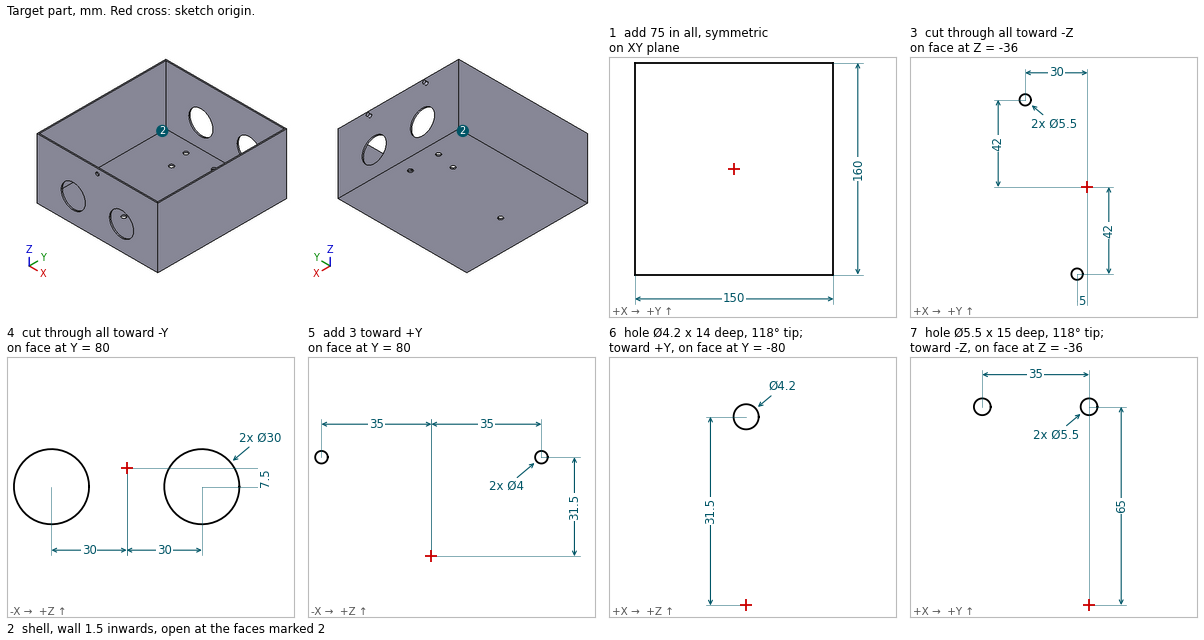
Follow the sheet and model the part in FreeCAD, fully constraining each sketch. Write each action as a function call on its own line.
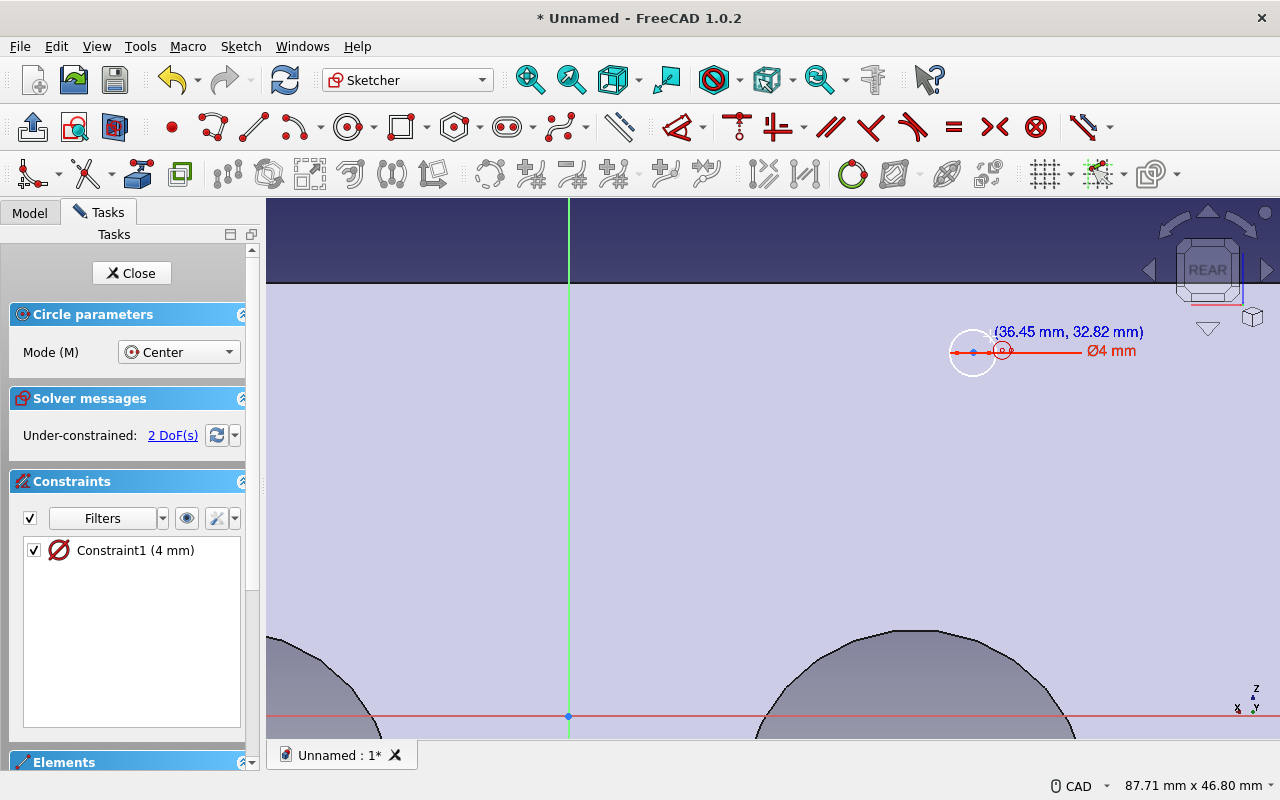
scroll(981, 358, down, 2)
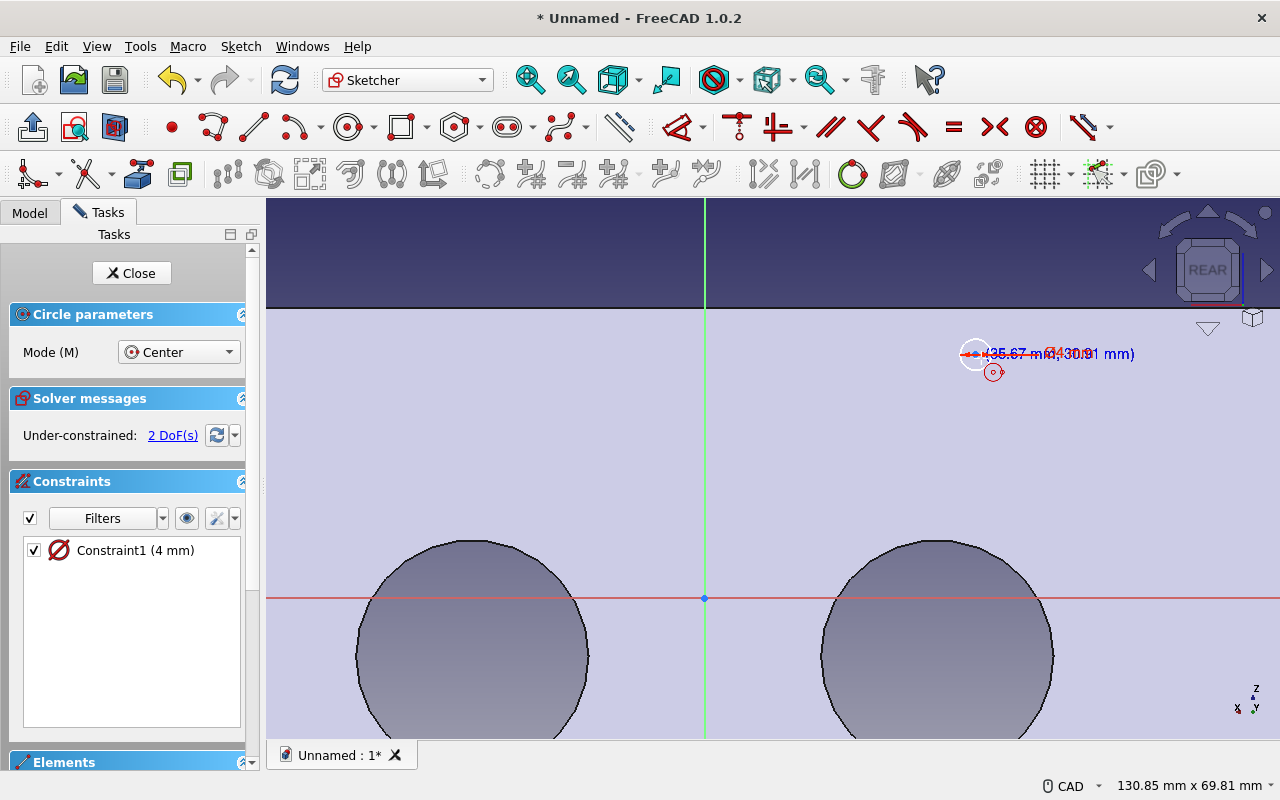
scroll(434, 354, up, 2)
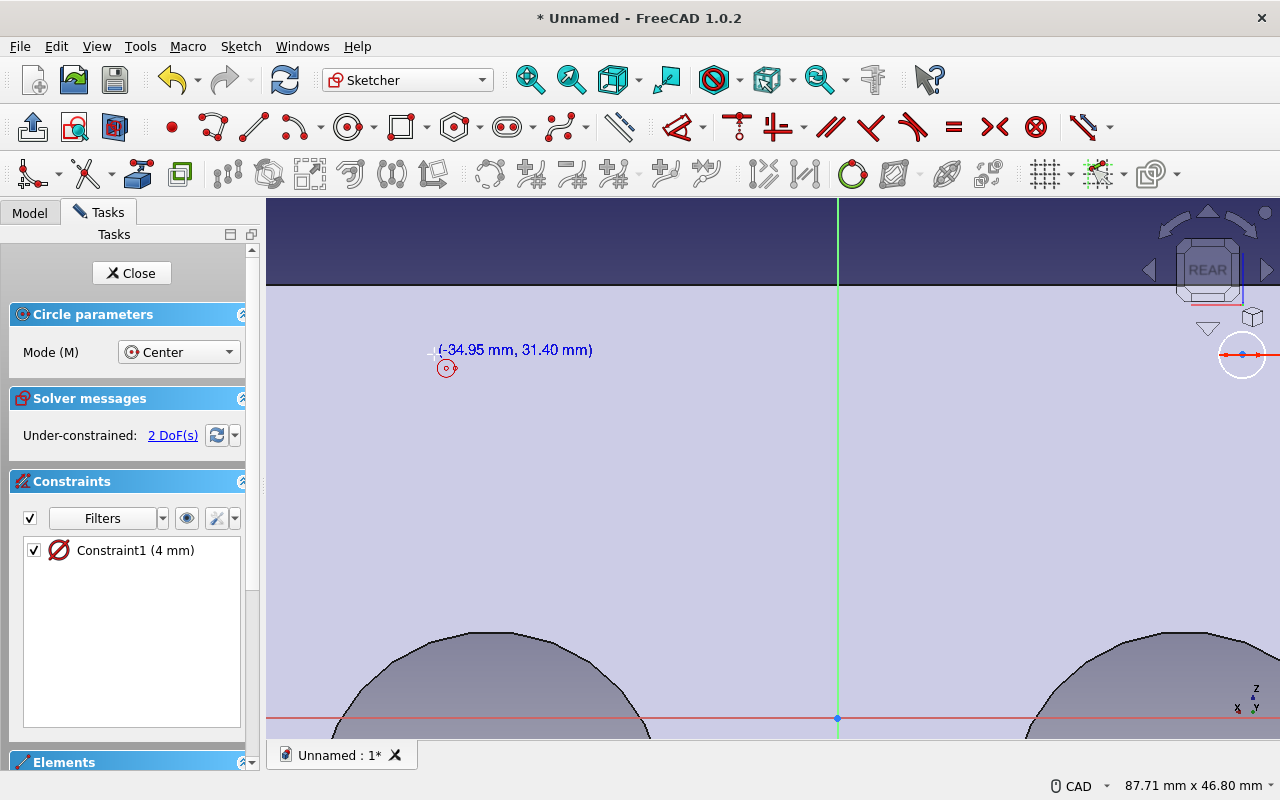
click(433, 354)
move(450, 338)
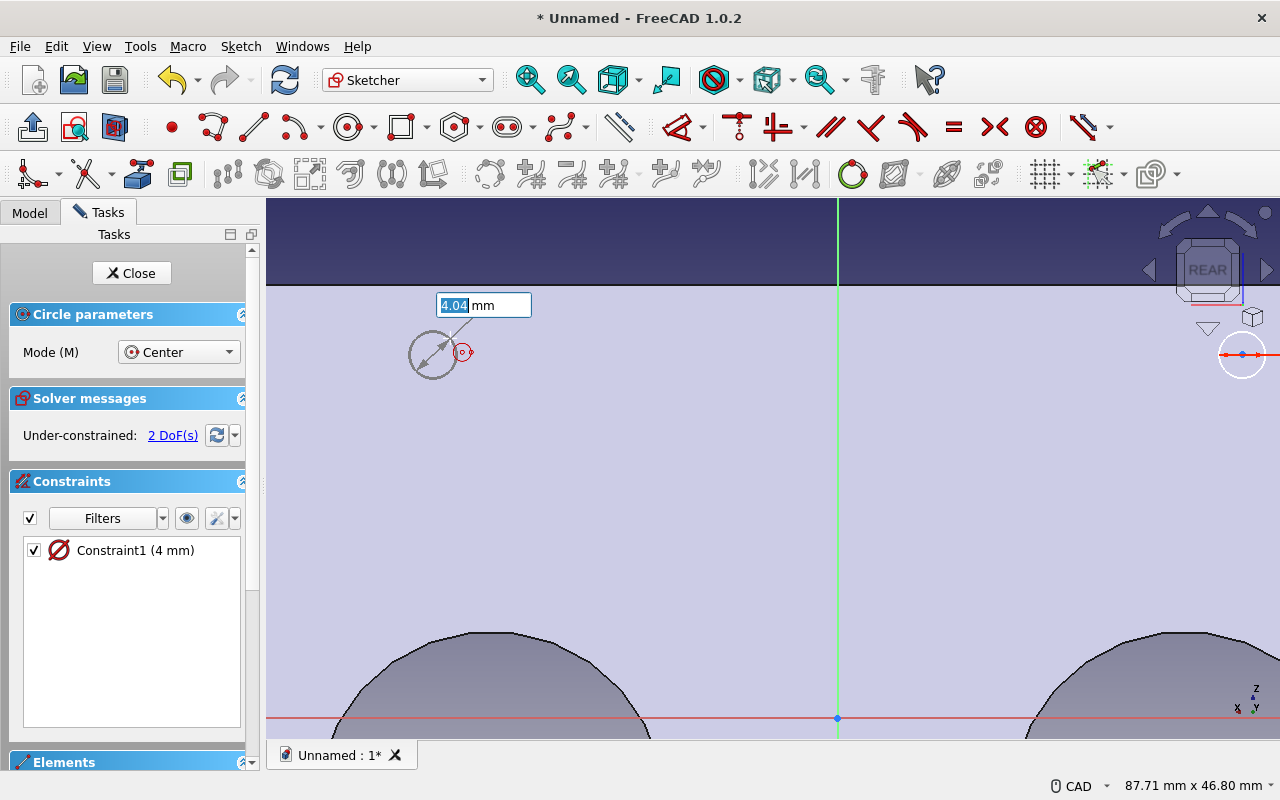
text(4)
key(Return)
key(Escape)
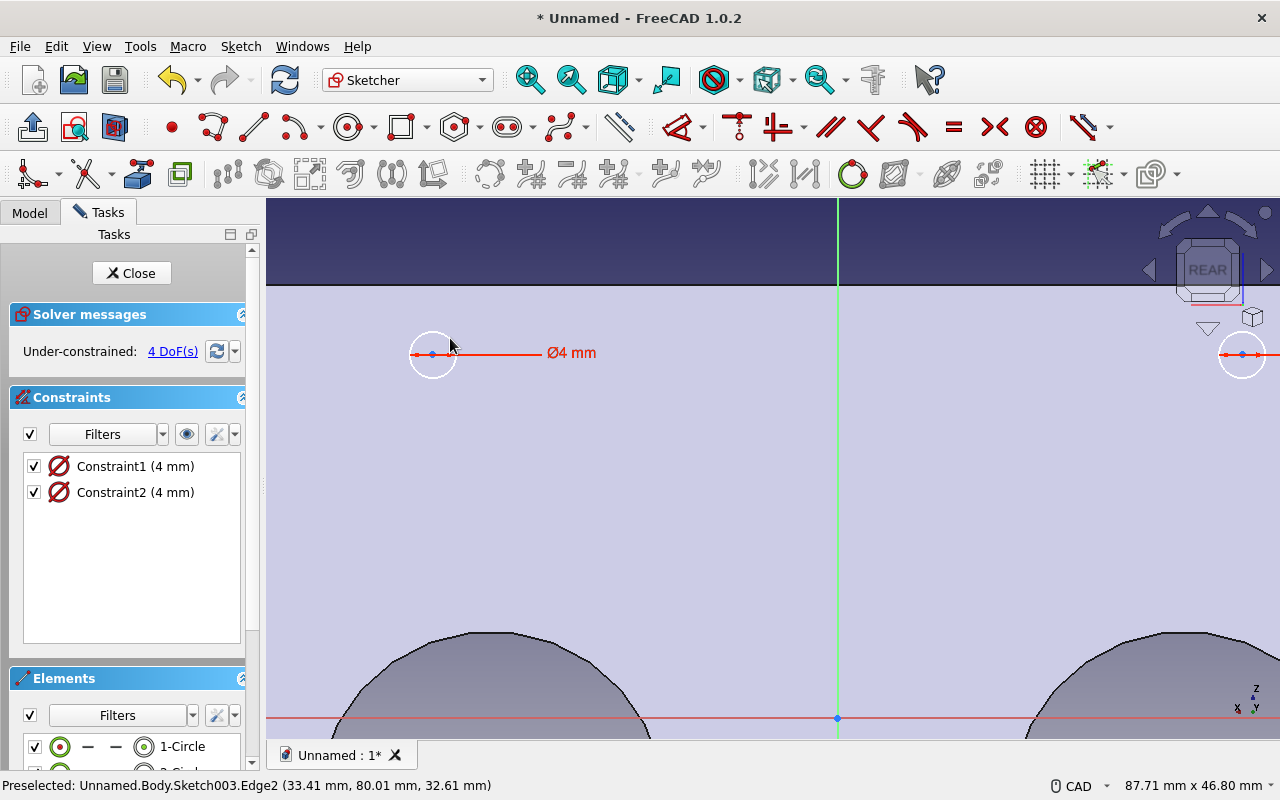
scroll(433, 354, down, 2)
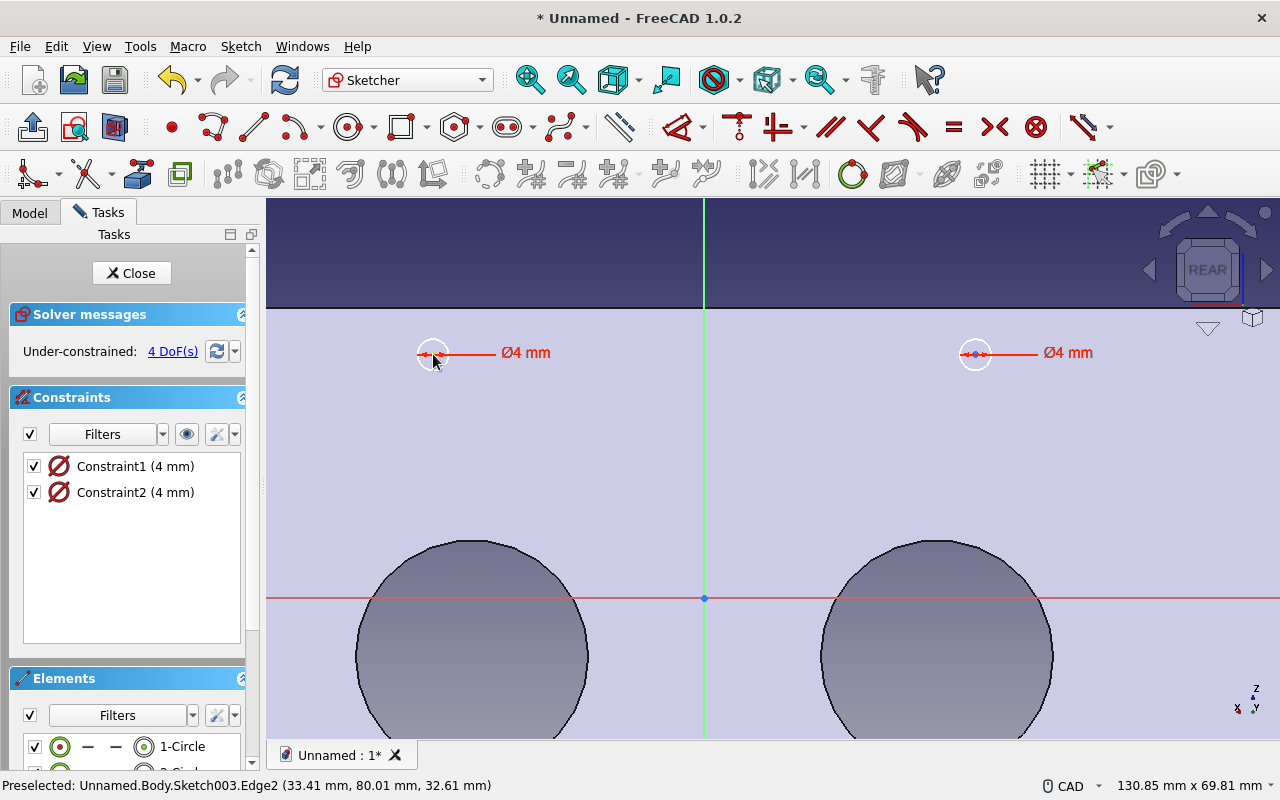
click(976, 355)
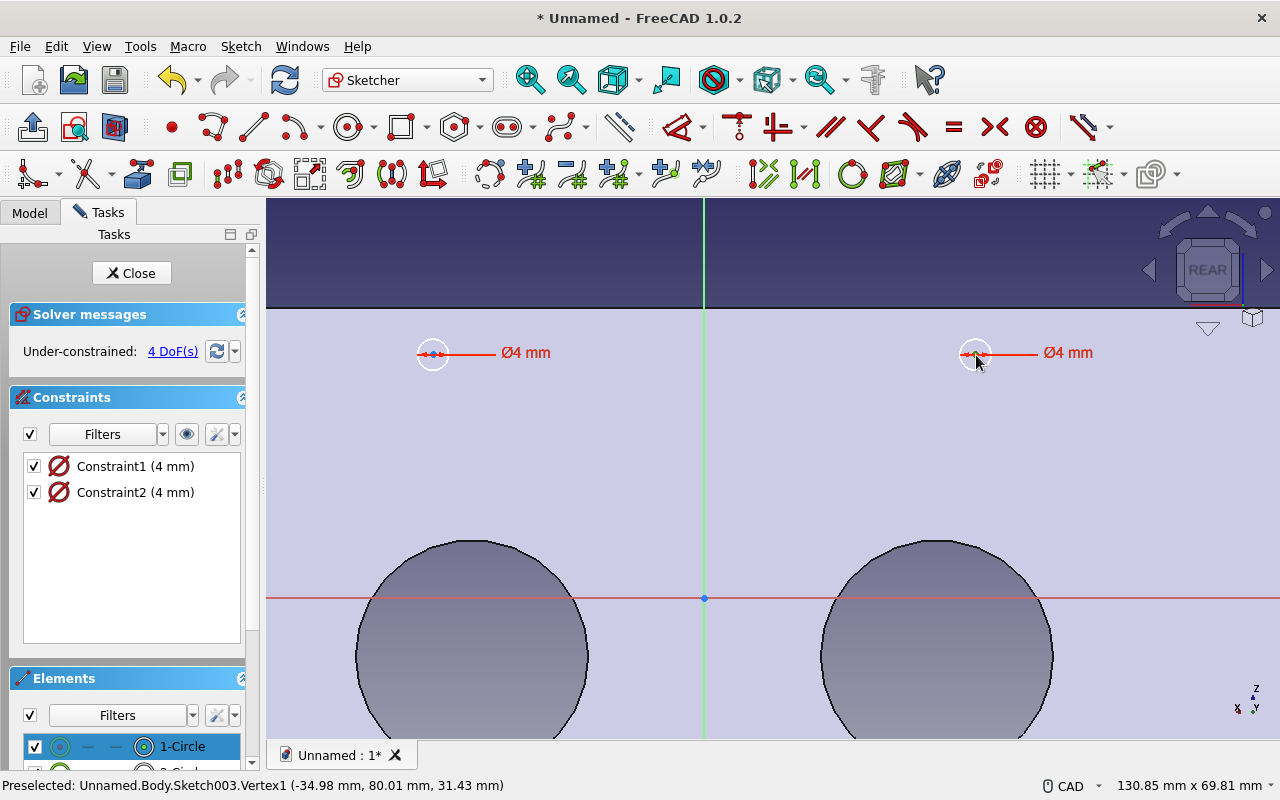
click(433, 355)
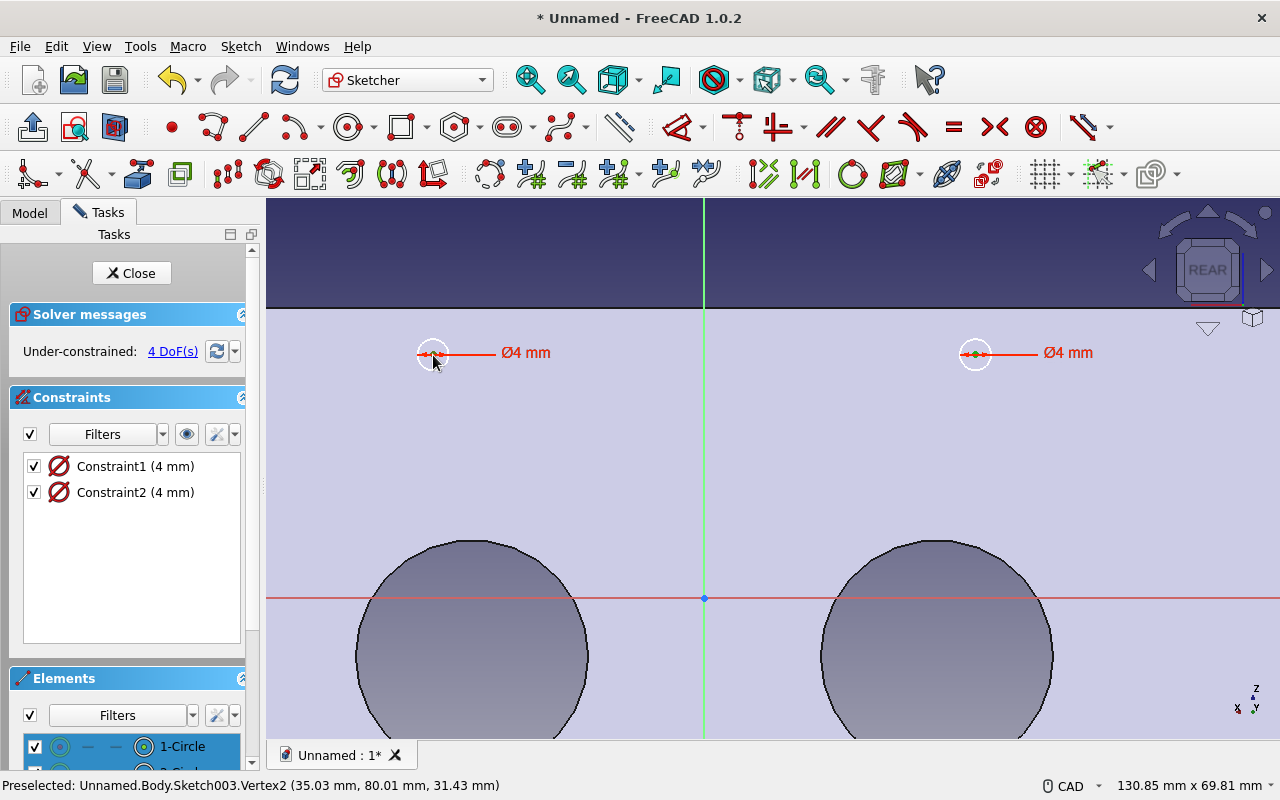
key(h)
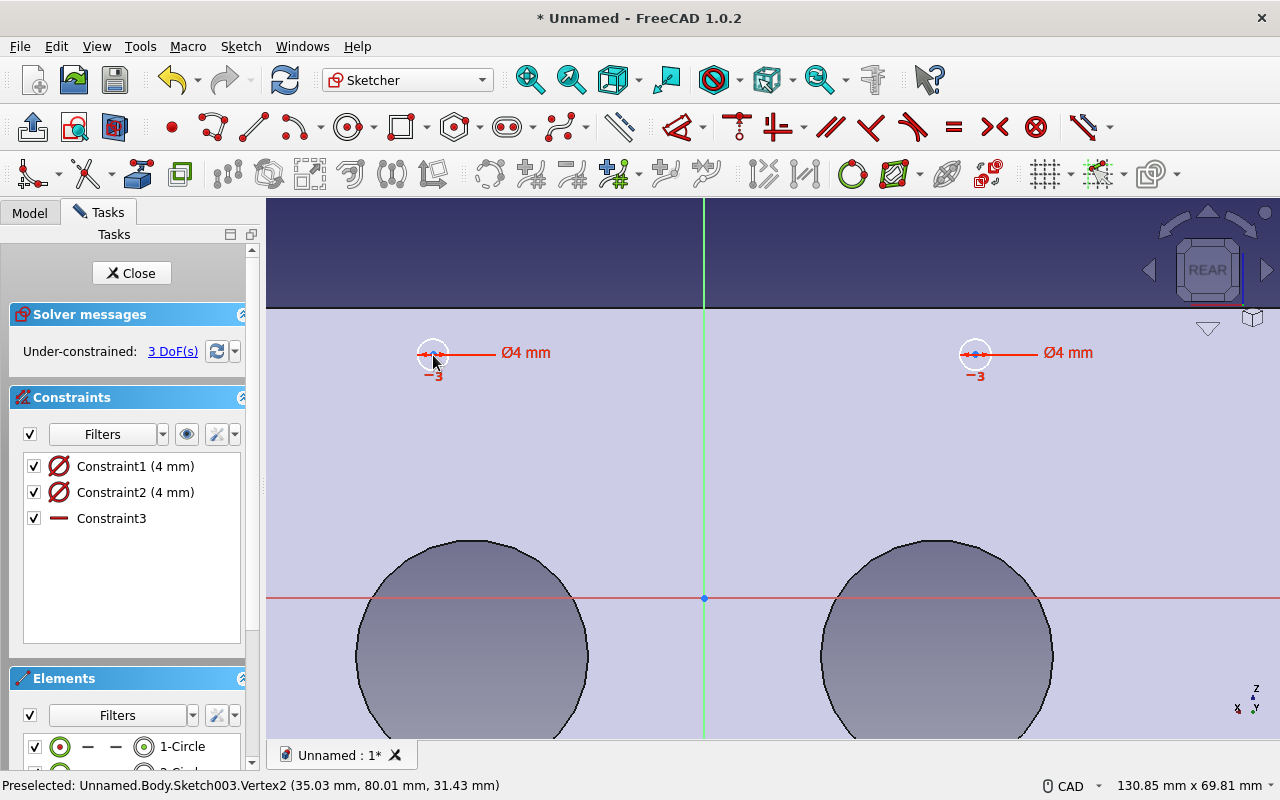
click(676, 128)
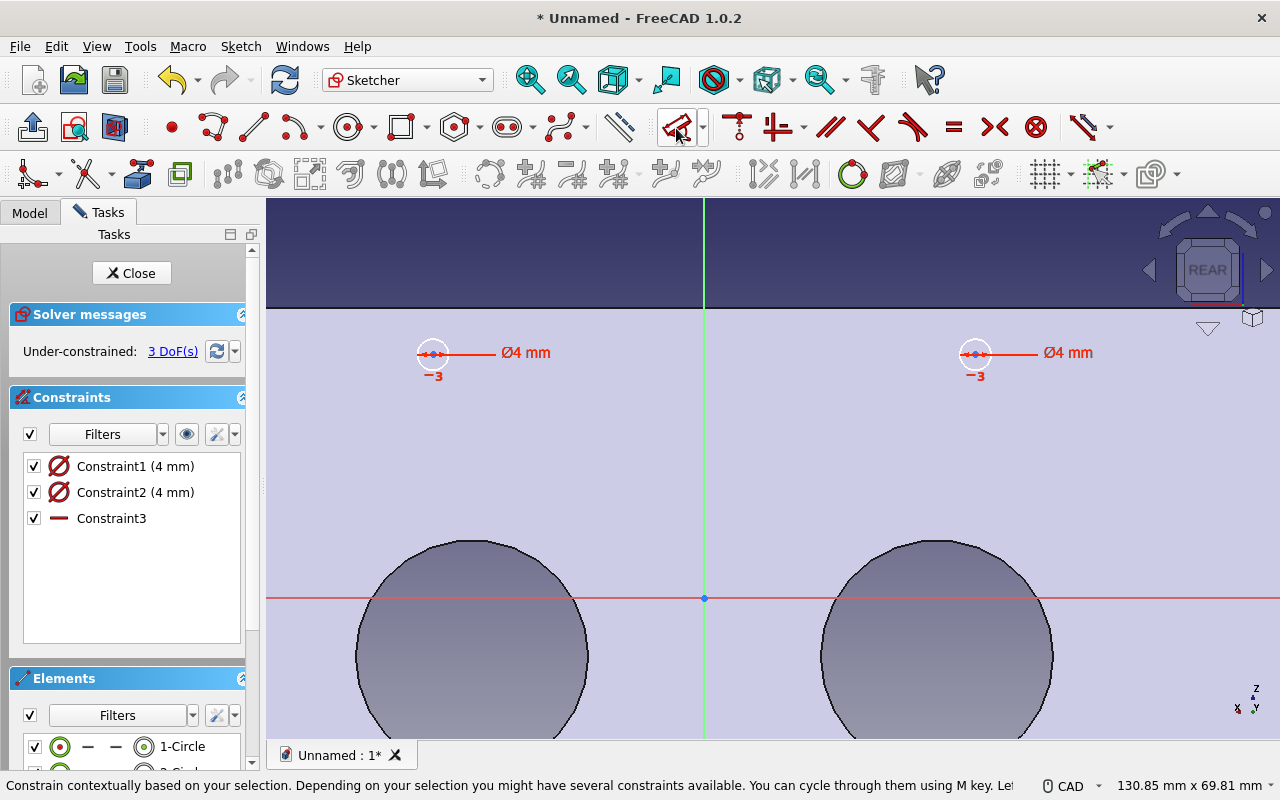
click(976, 355)
click(840, 632)